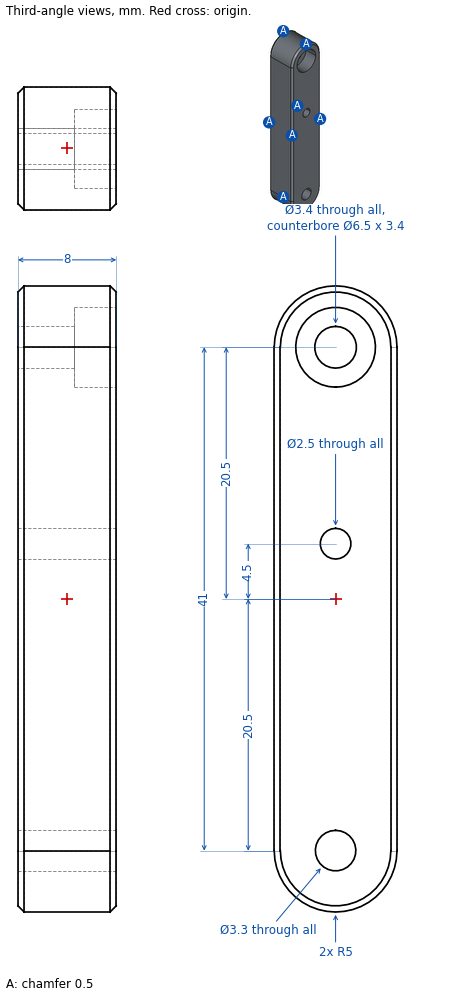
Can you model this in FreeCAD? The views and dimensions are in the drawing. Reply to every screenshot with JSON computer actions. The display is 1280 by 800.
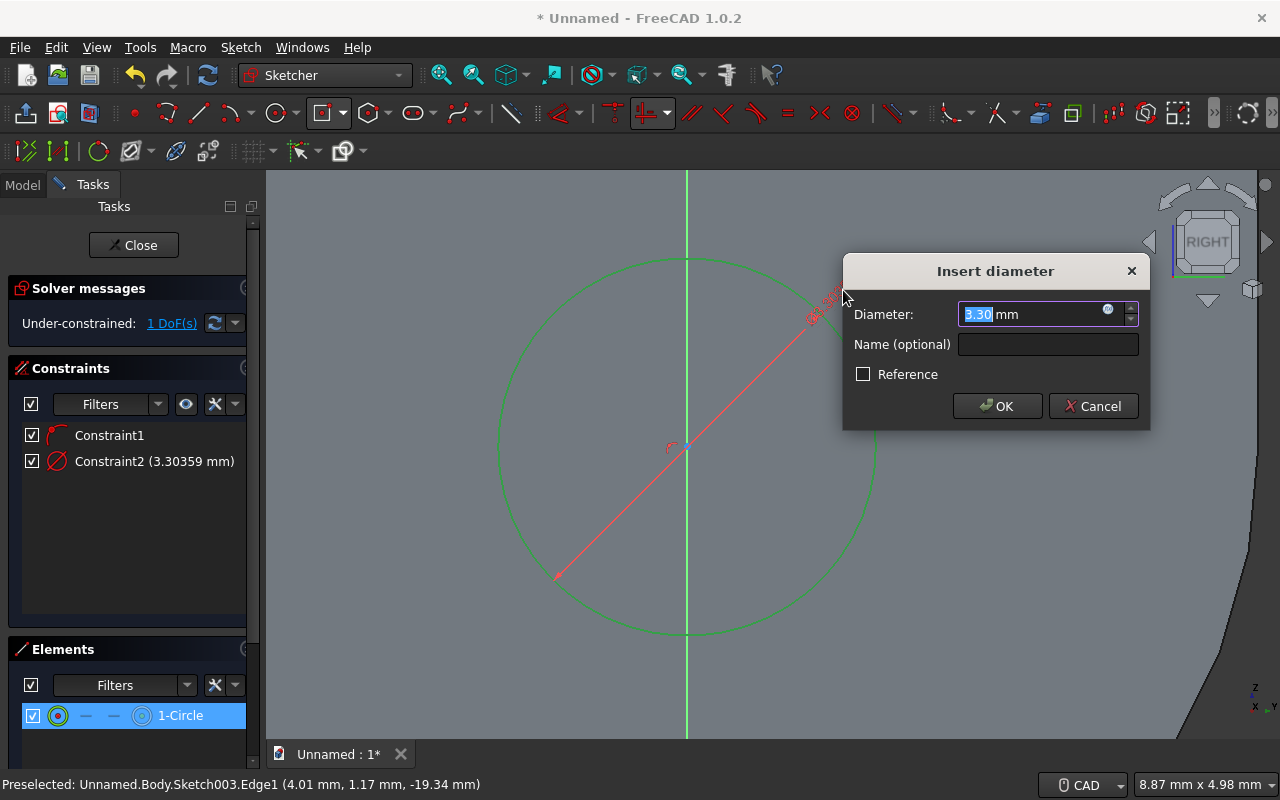
{"action": "type", "text": "3.3"}
{"action": "key", "text": "Return"}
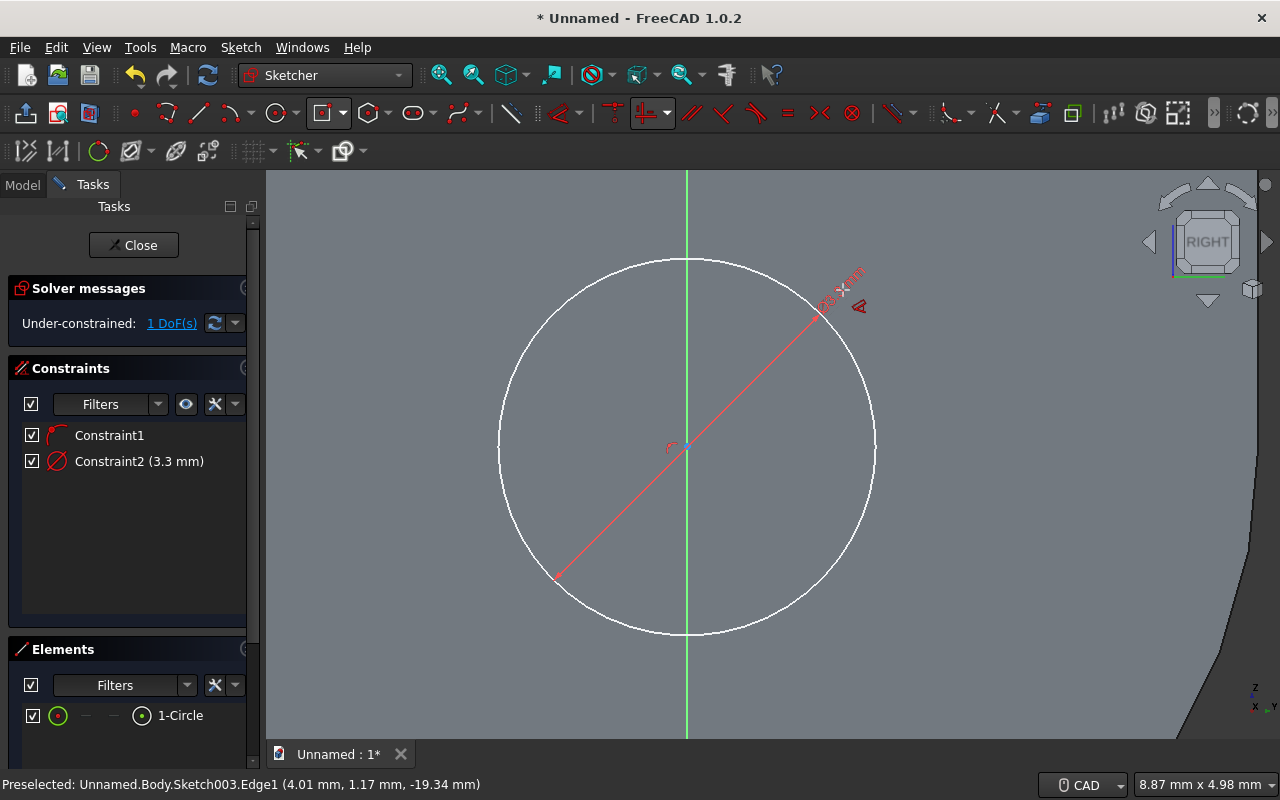
{"action": "left_click", "coordinate": [687, 447]}
{"action": "left_click", "coordinate": [721, 322]}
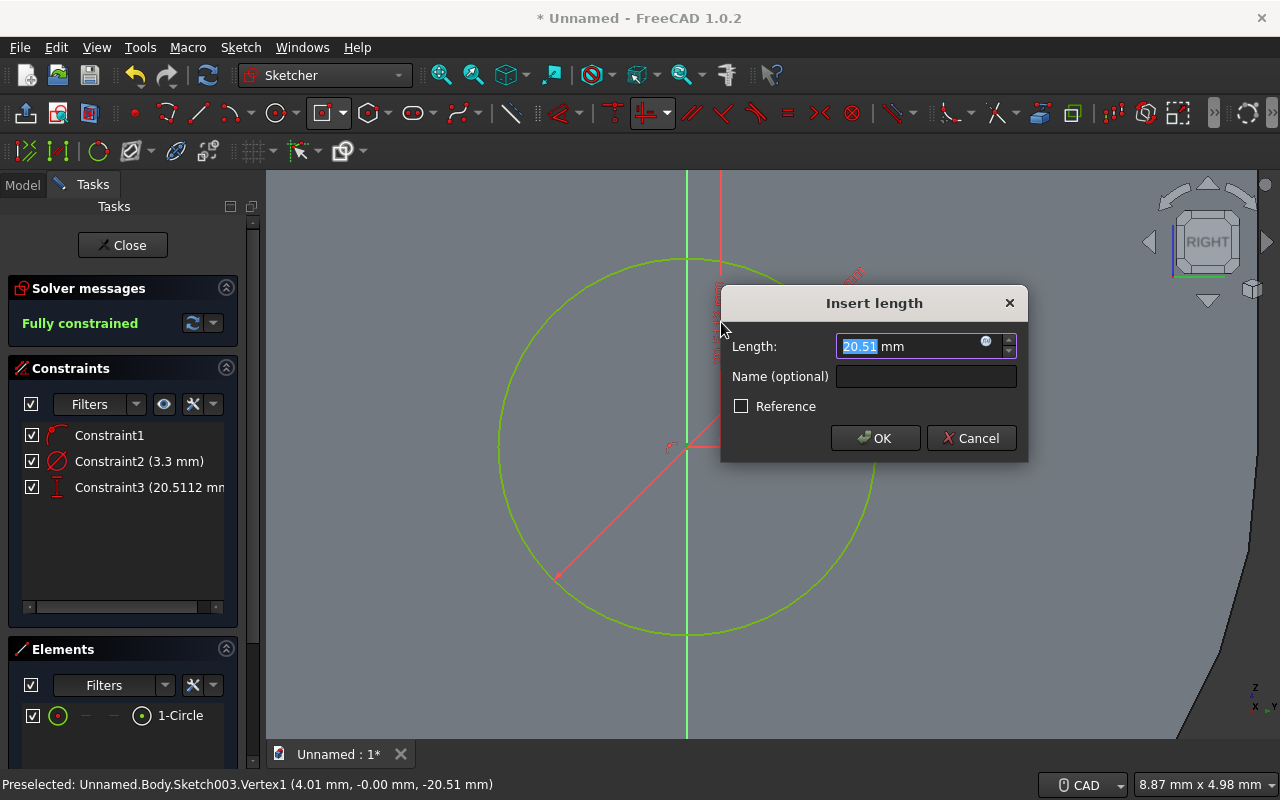
{"action": "type", "text": "20.5"}
{"action": "key", "text": "Return"}
{"action": "key", "text": "Escape"}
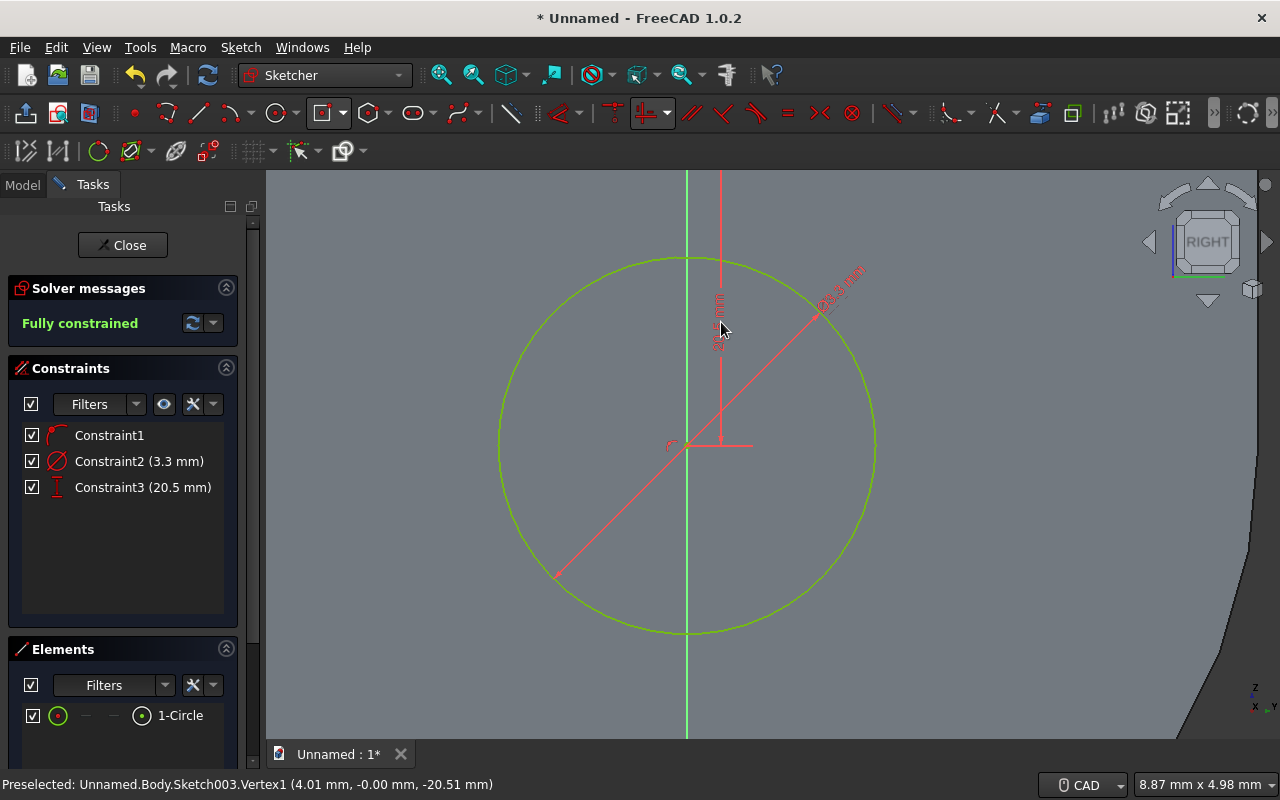
{"action": "left_click", "coordinate": [123, 245]}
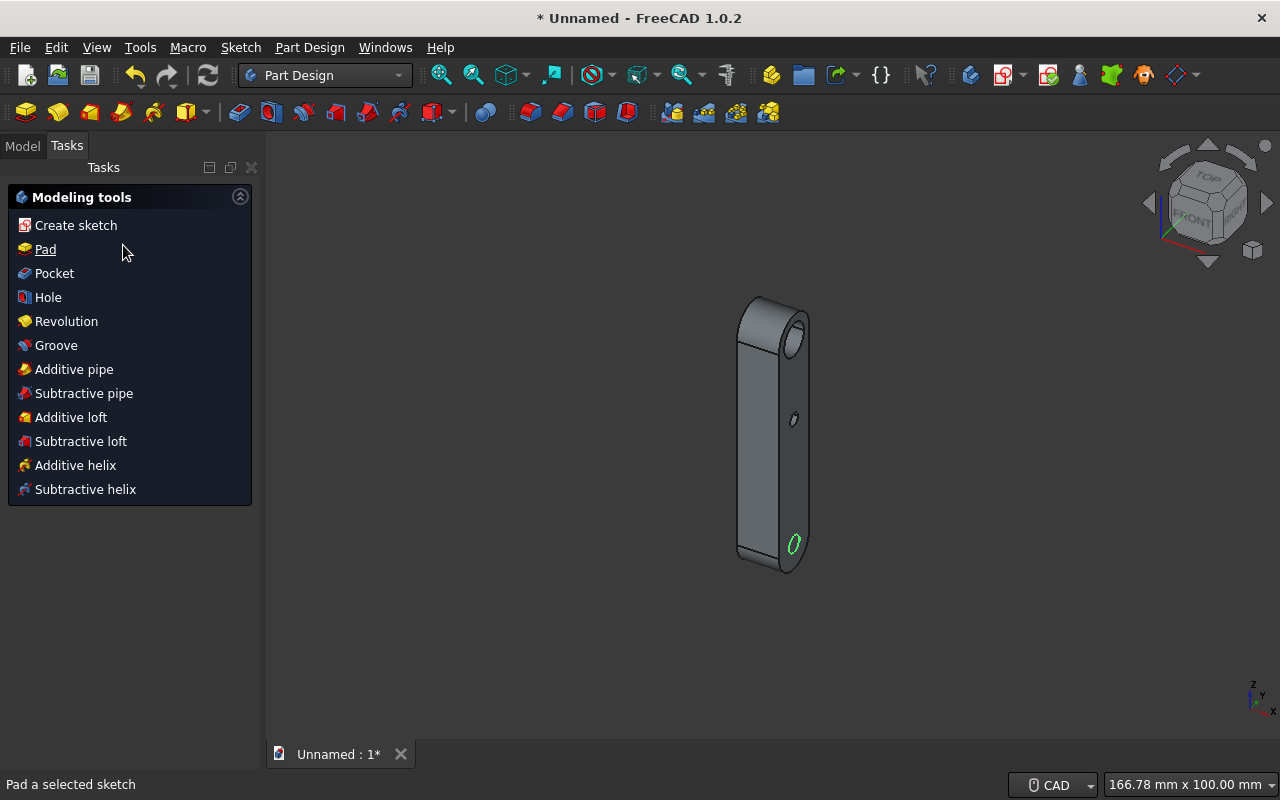
{"action": "left_click", "coordinate": [272, 112]}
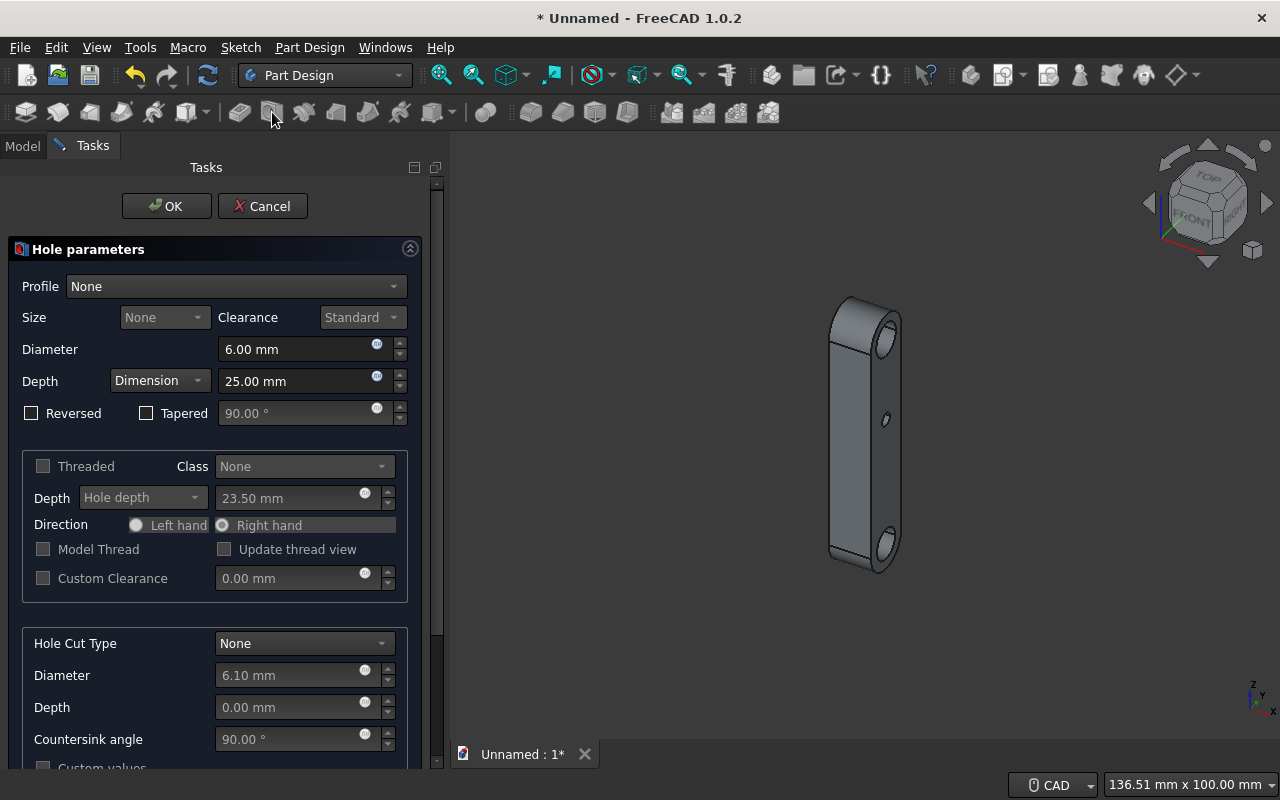
{"action": "triple_click", "coordinate": [305, 349]}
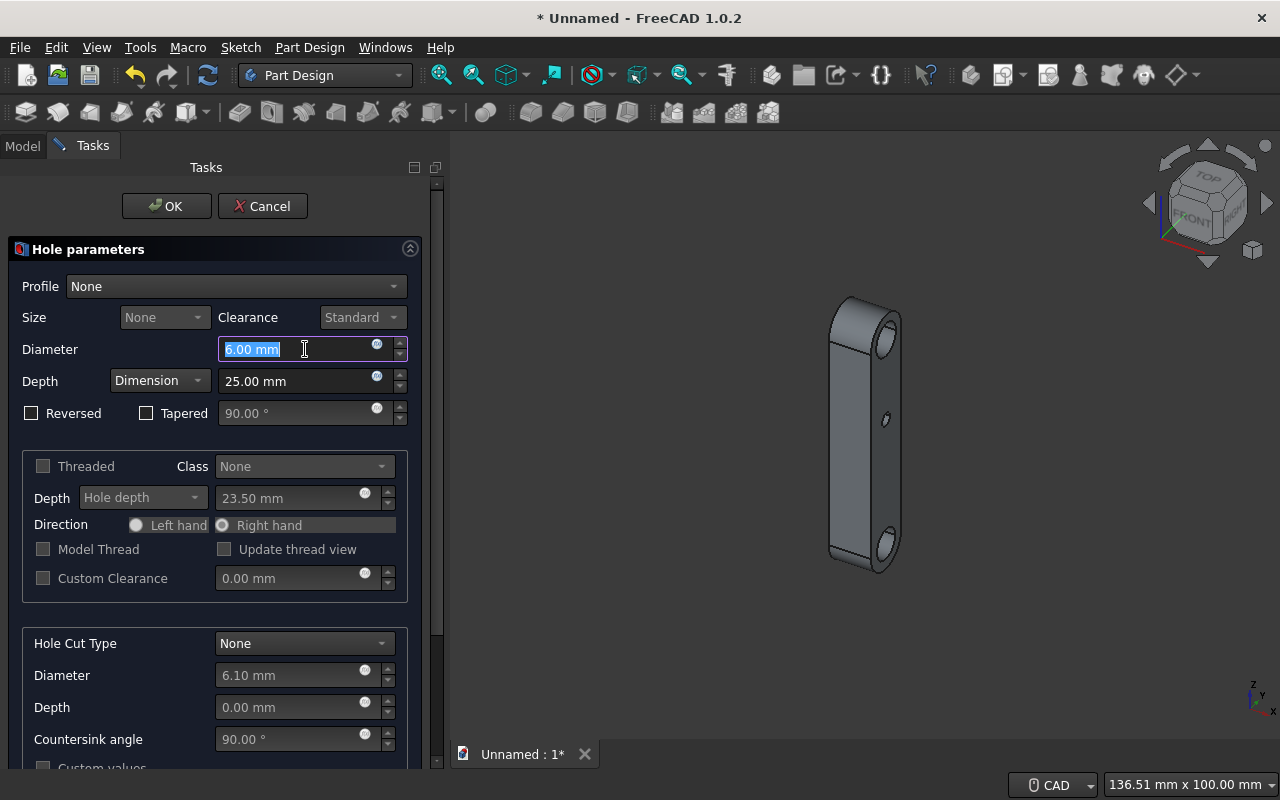
{"action": "type", "text": "3.3"}
{"action": "key", "text": "Tab"}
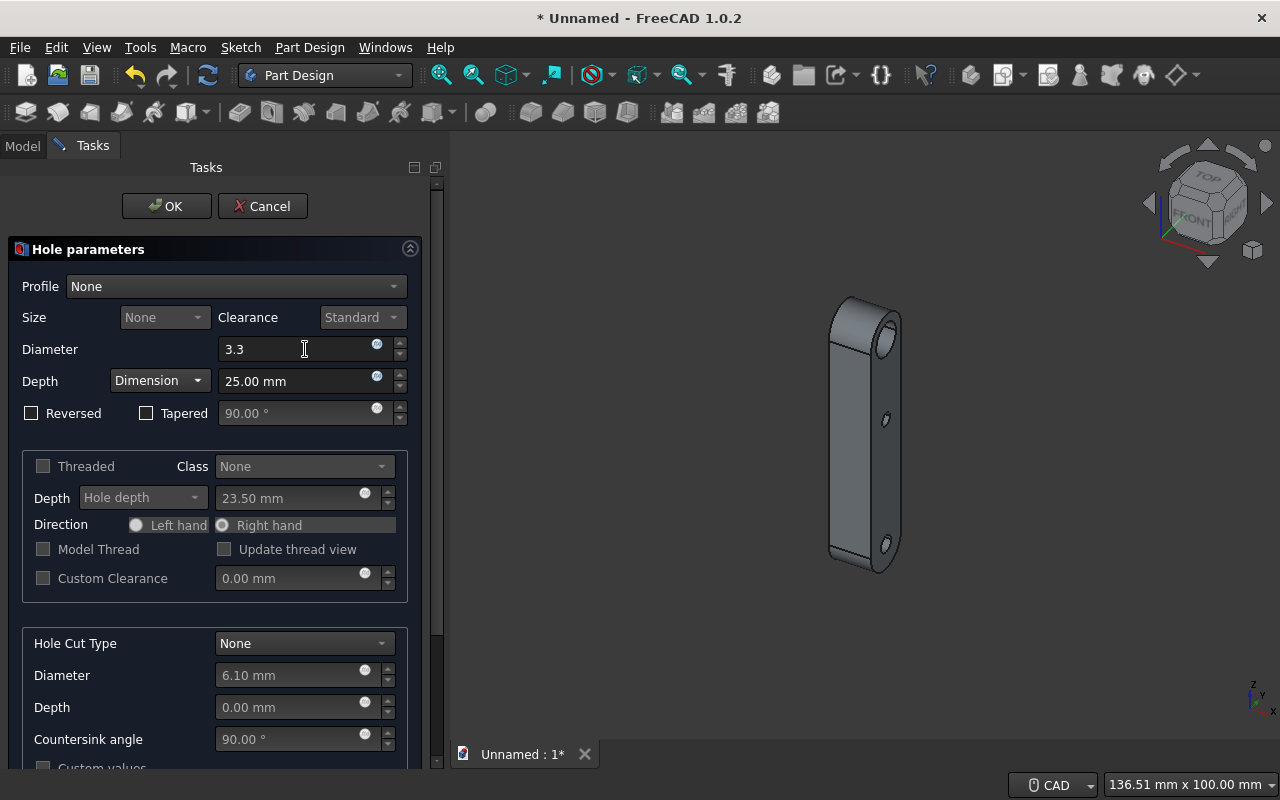
{"action": "left_click", "coordinate": [161, 380]}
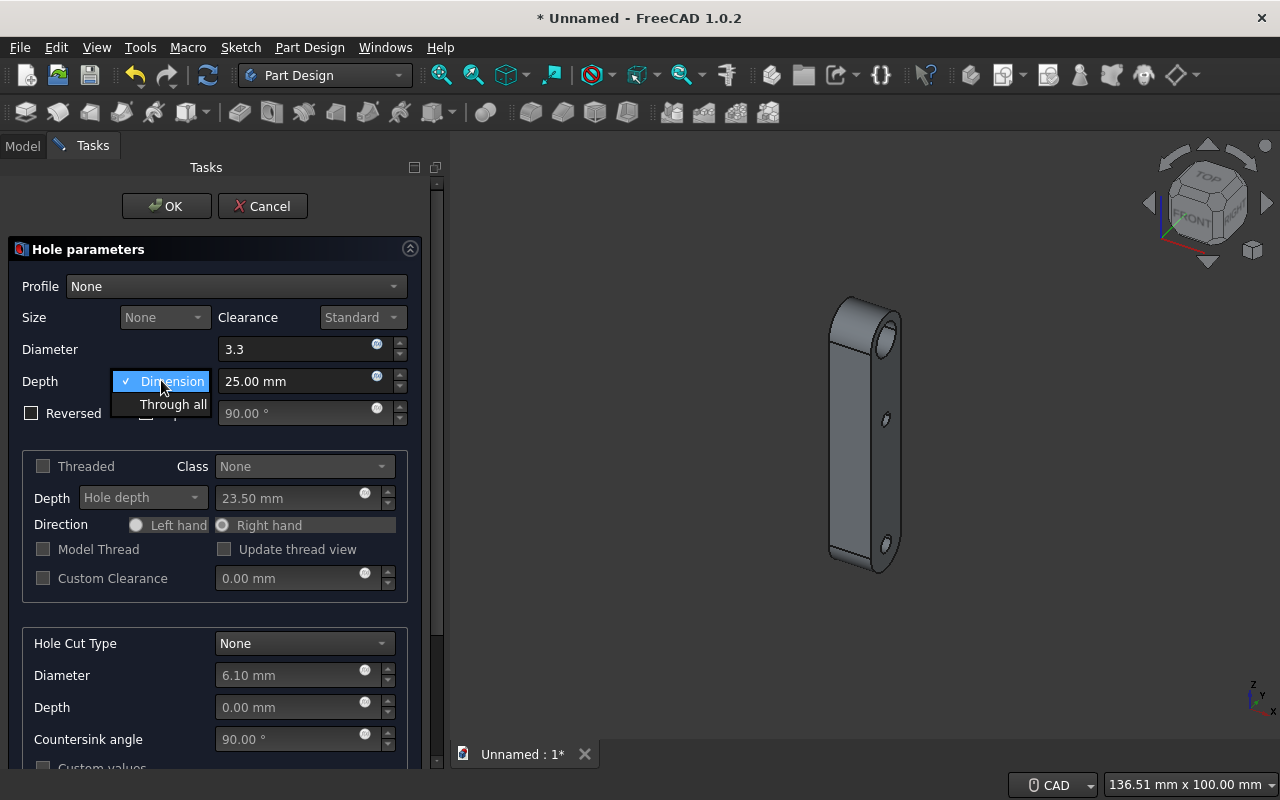
{"action": "left_click", "coordinate": [160, 404]}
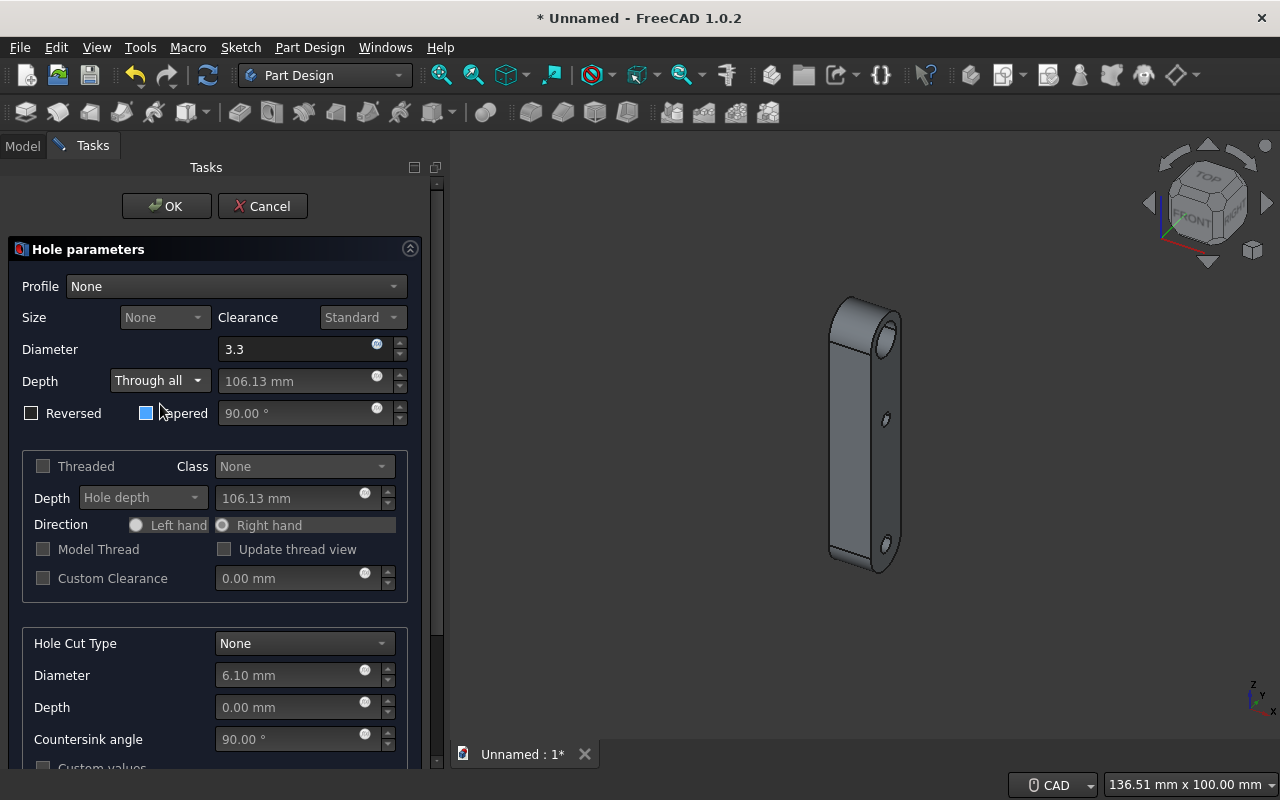
{"action": "left_click", "coordinate": [167, 206]}